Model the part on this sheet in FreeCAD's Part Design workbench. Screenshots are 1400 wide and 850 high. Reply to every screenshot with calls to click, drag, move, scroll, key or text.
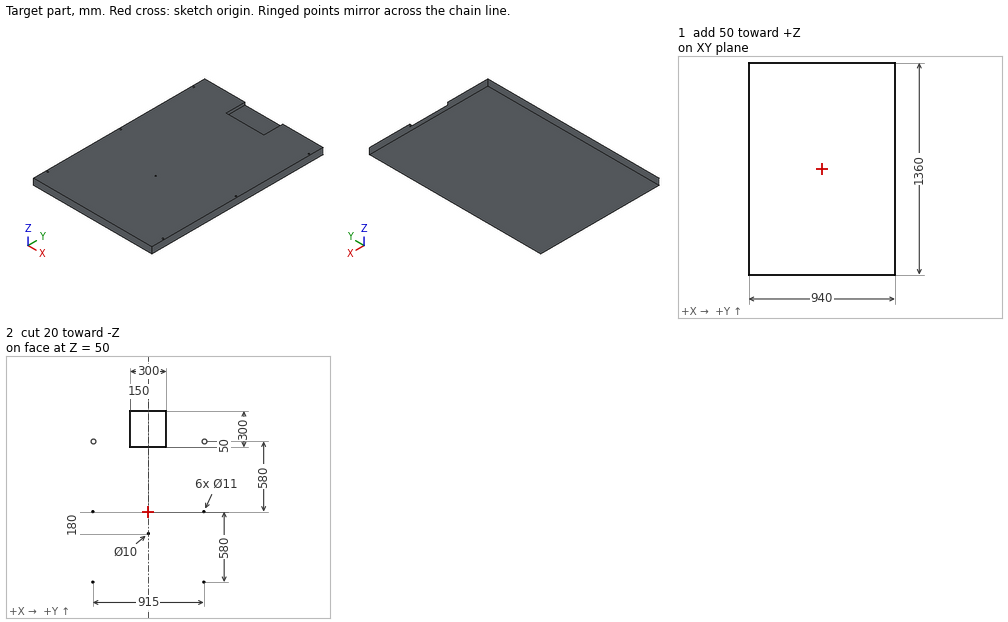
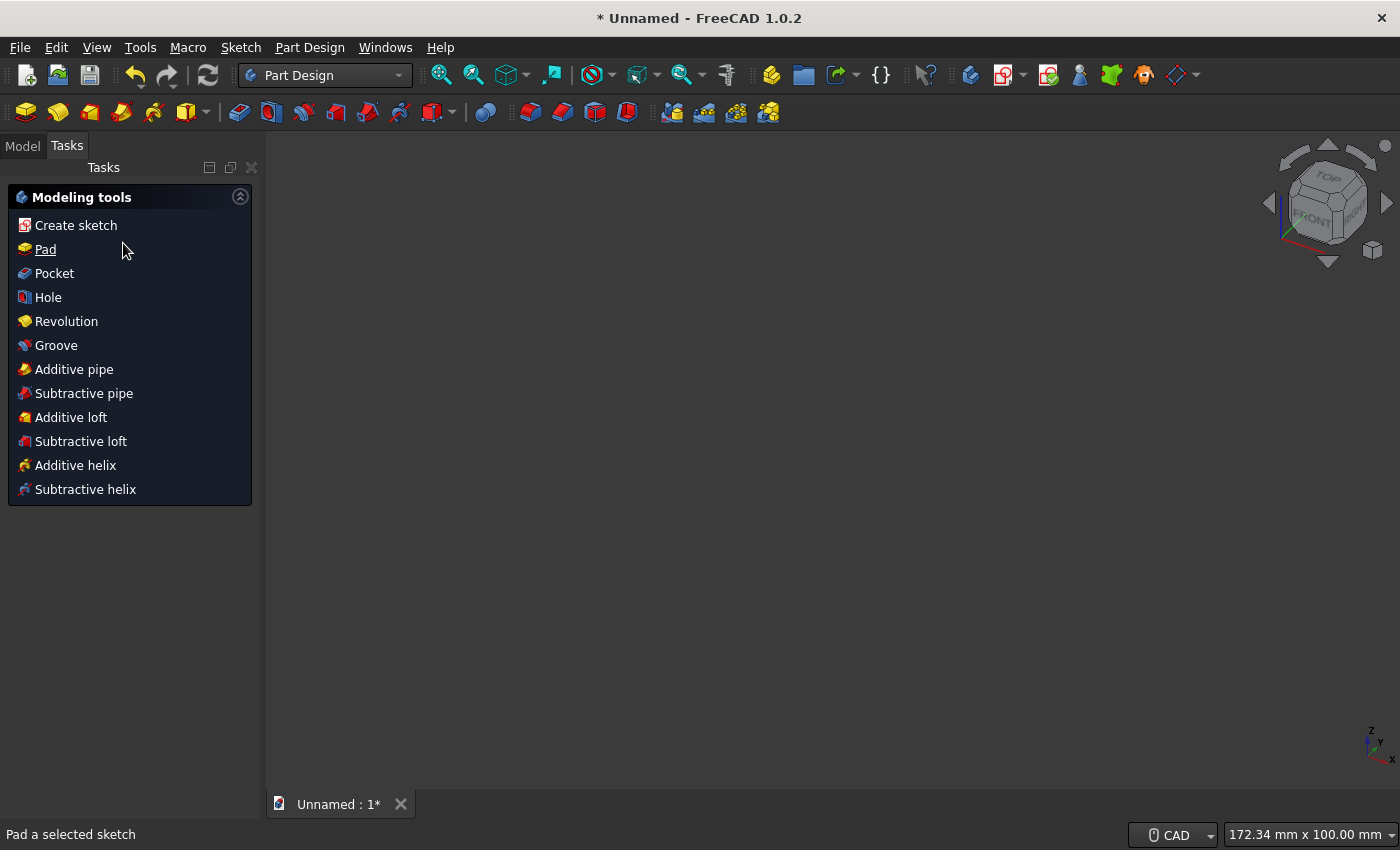
click(26, 112)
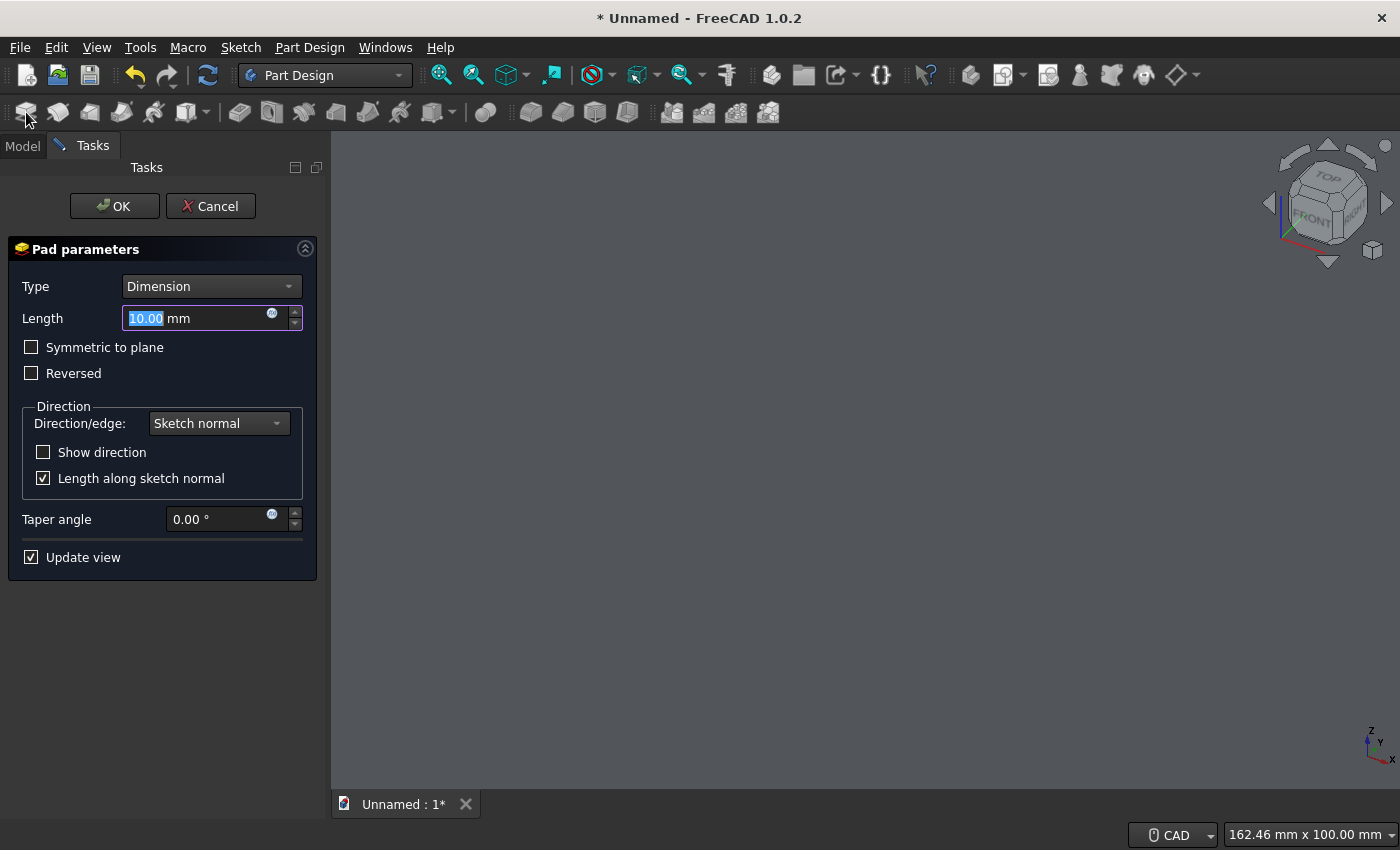
text(50)
key(Tab)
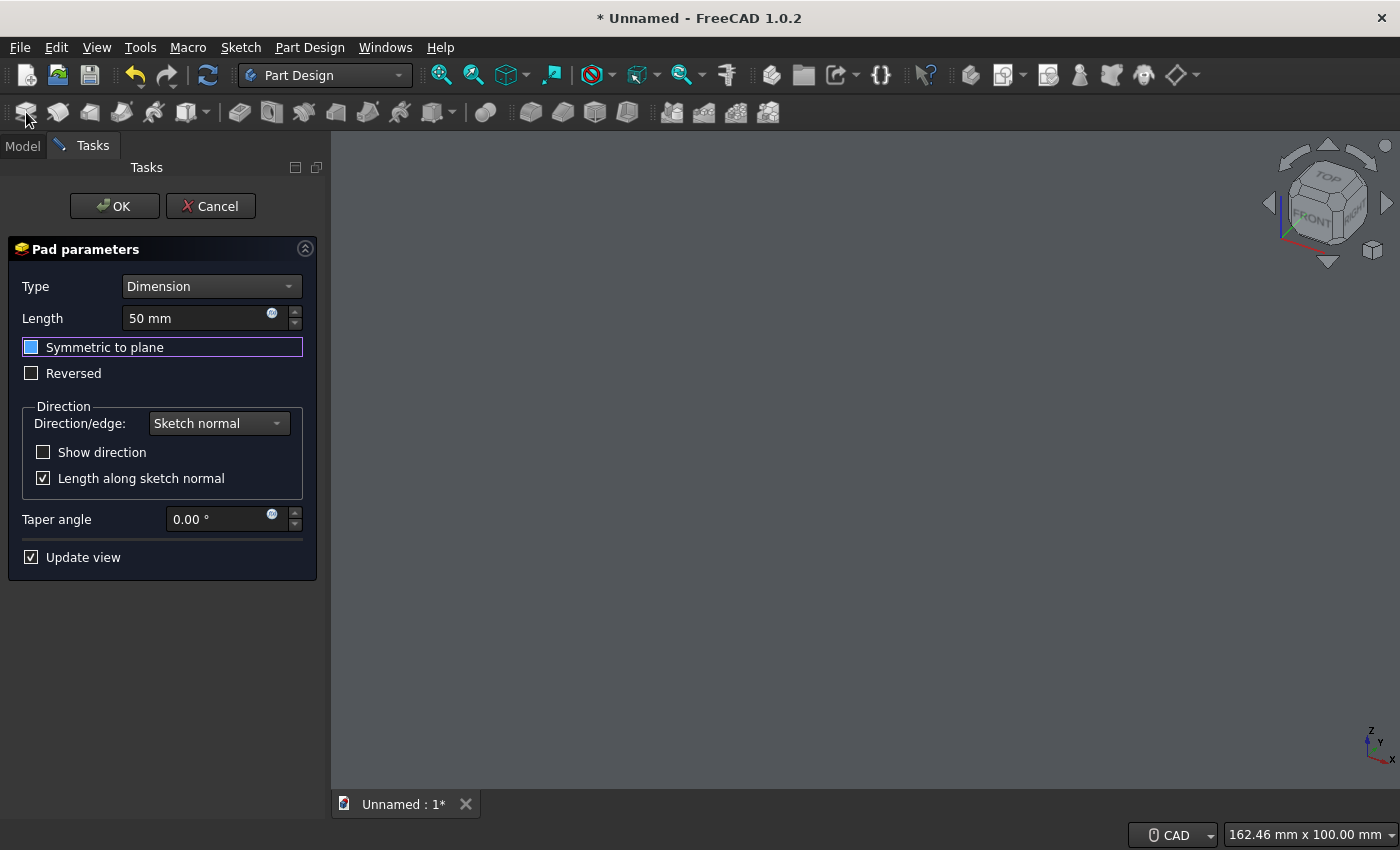
click(115, 206)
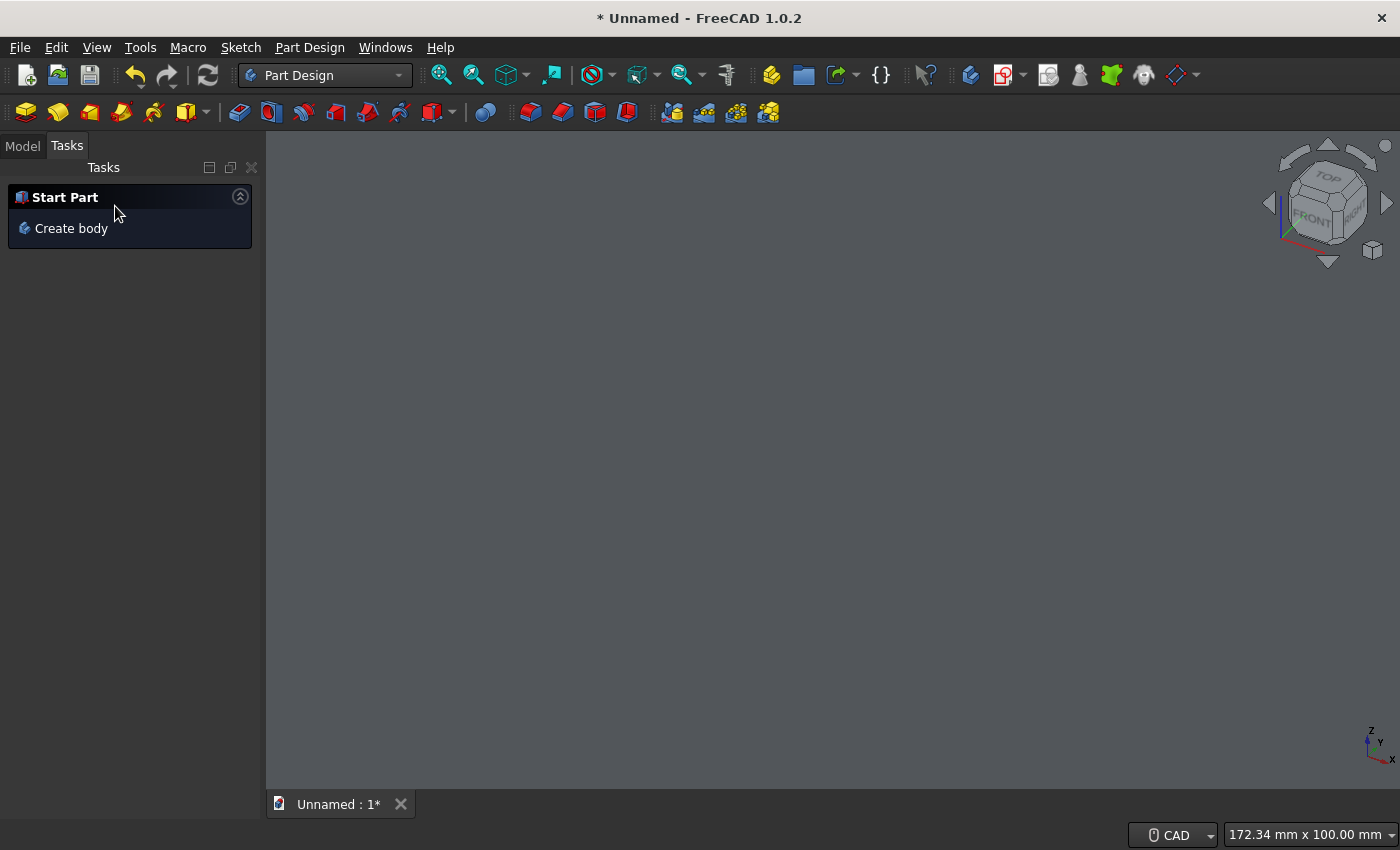
key(v)
key(f)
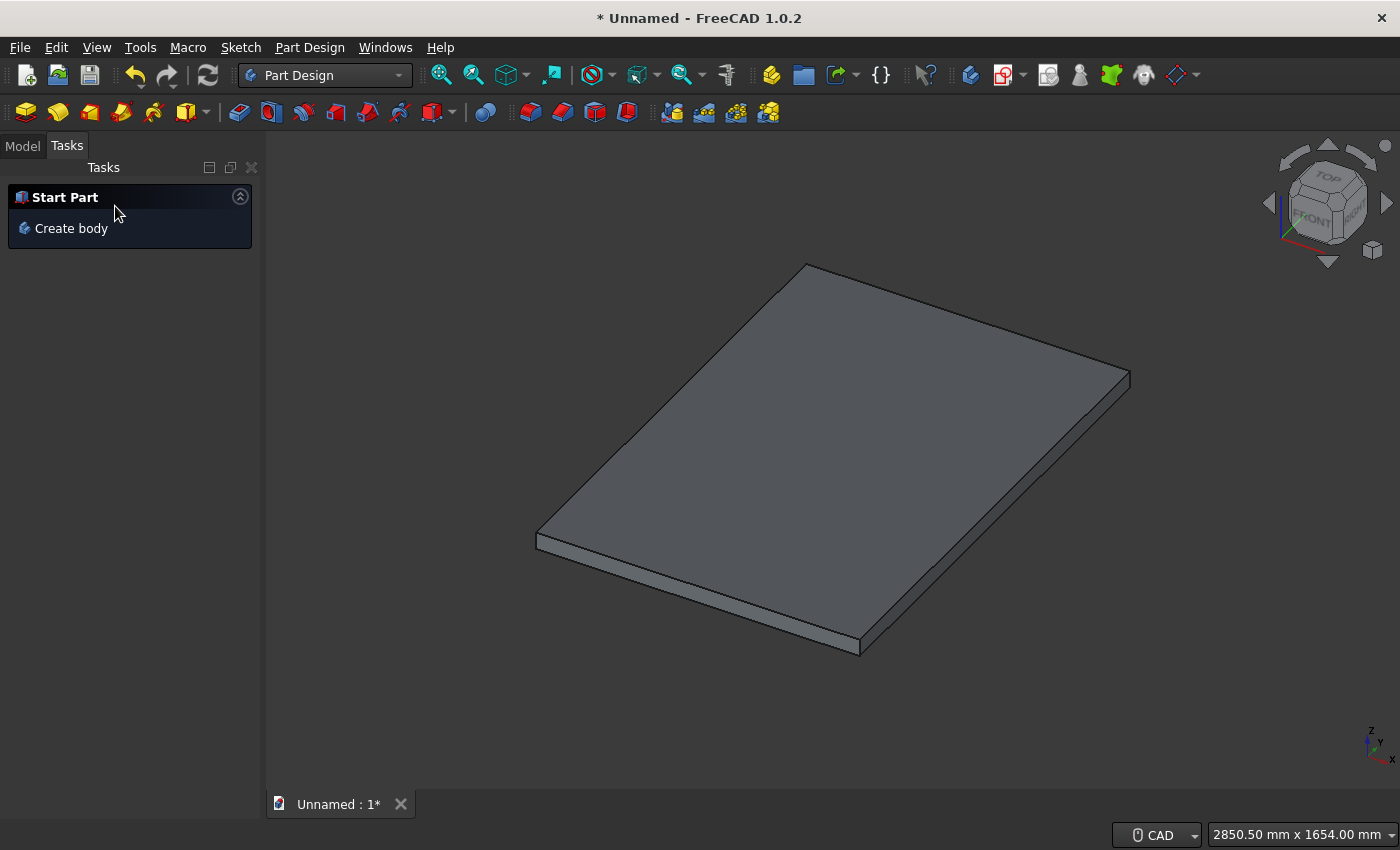
click(872, 412)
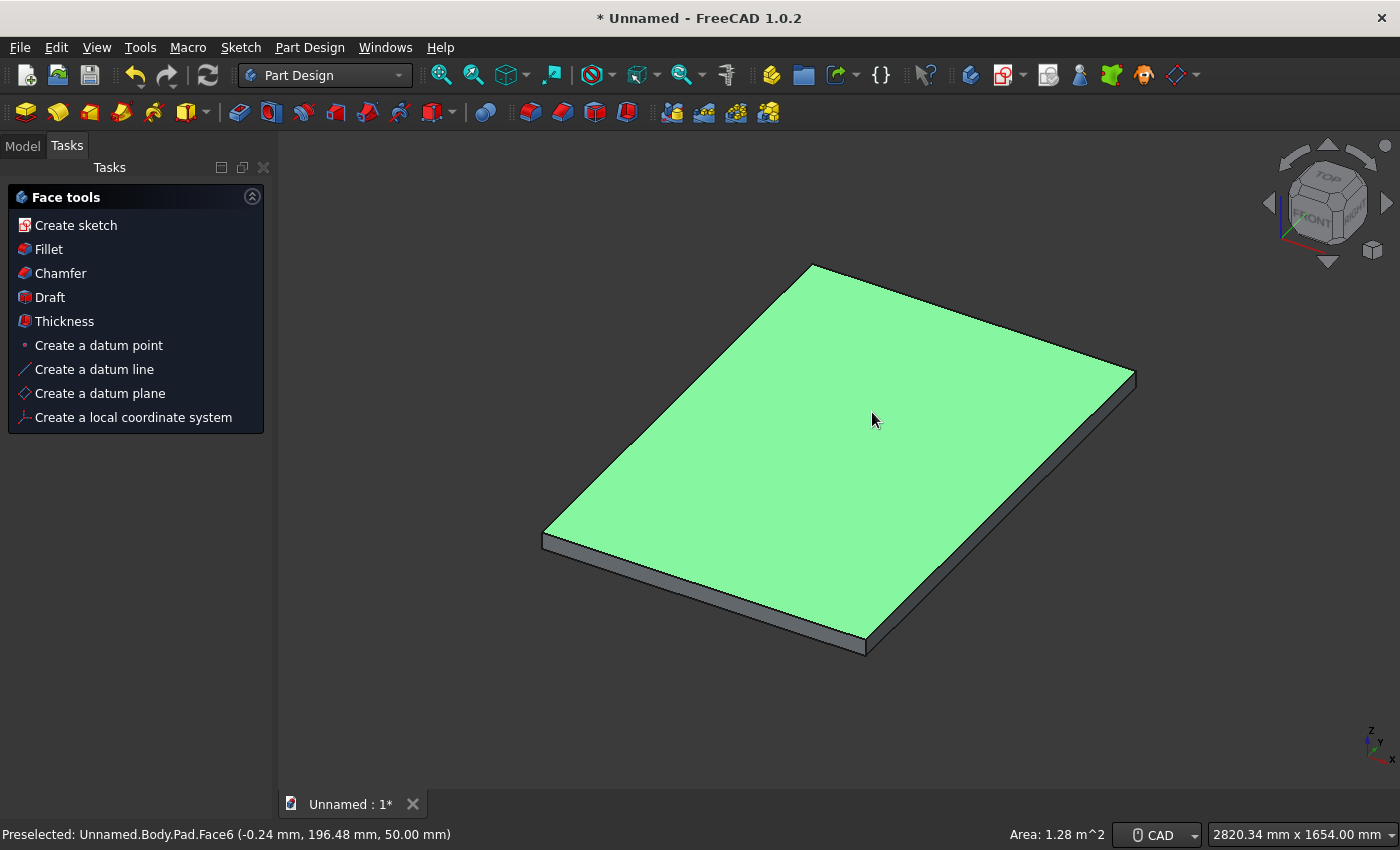
click(1004, 76)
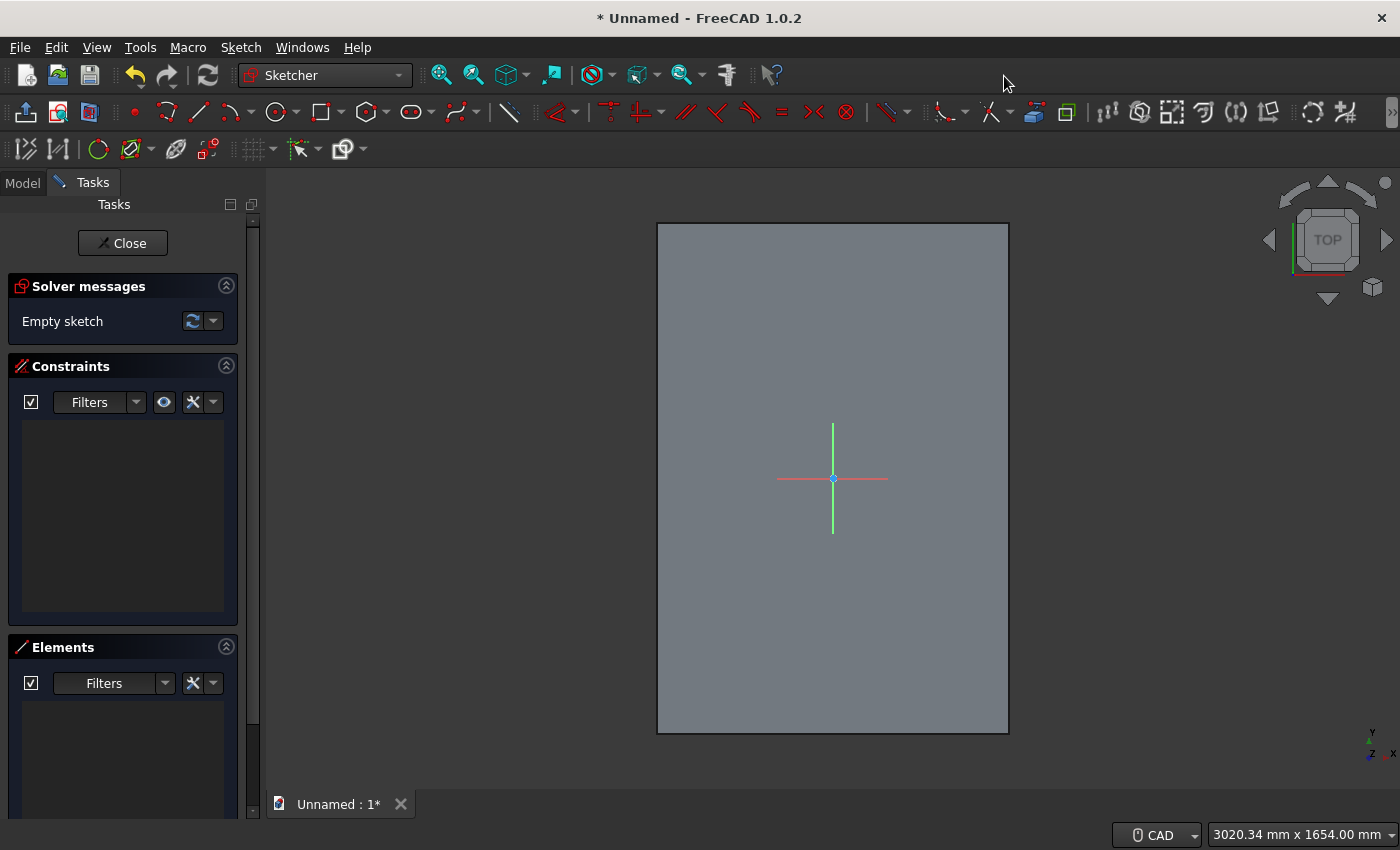
scroll(455, 686, down, 1)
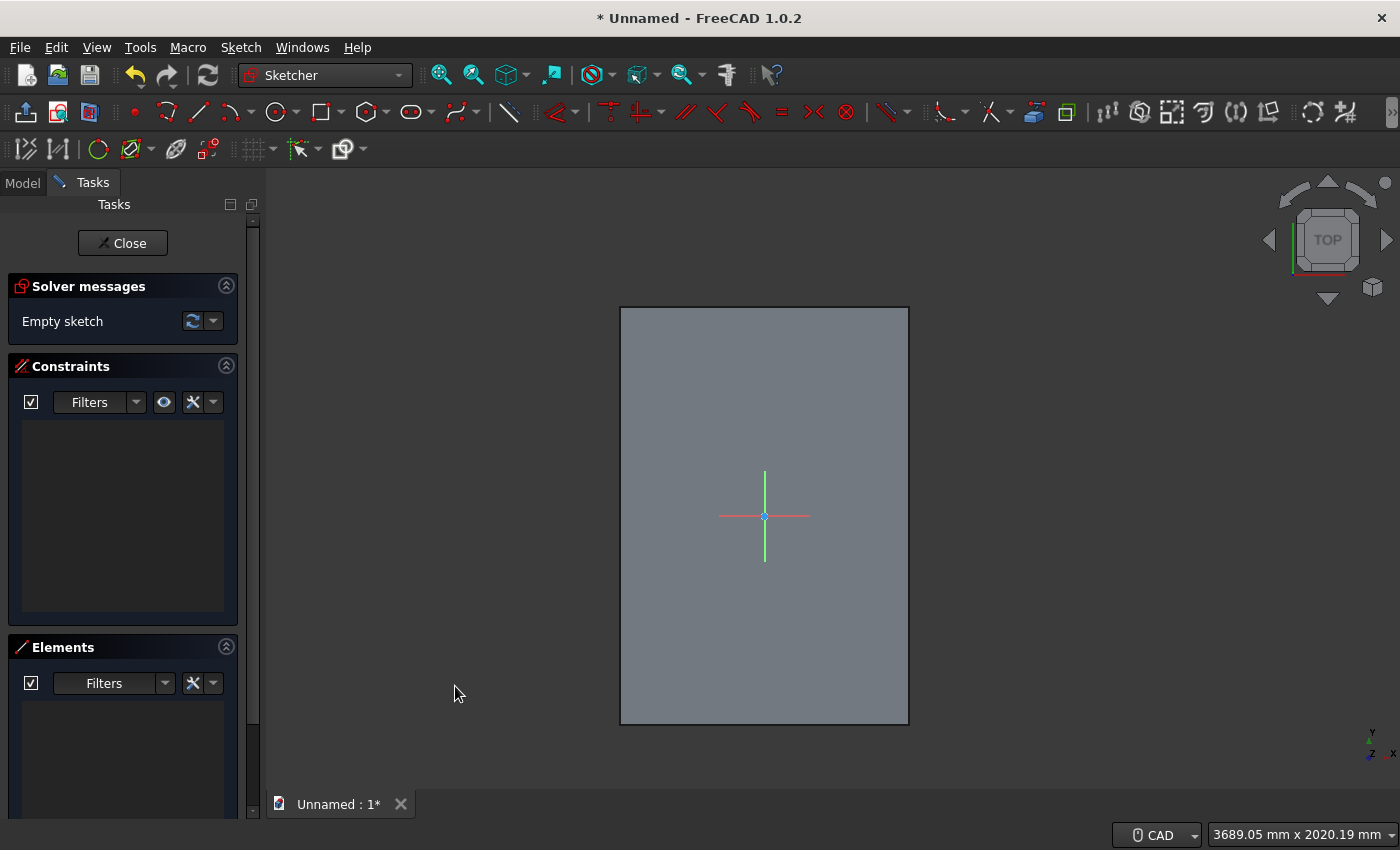
key(g)
key(r)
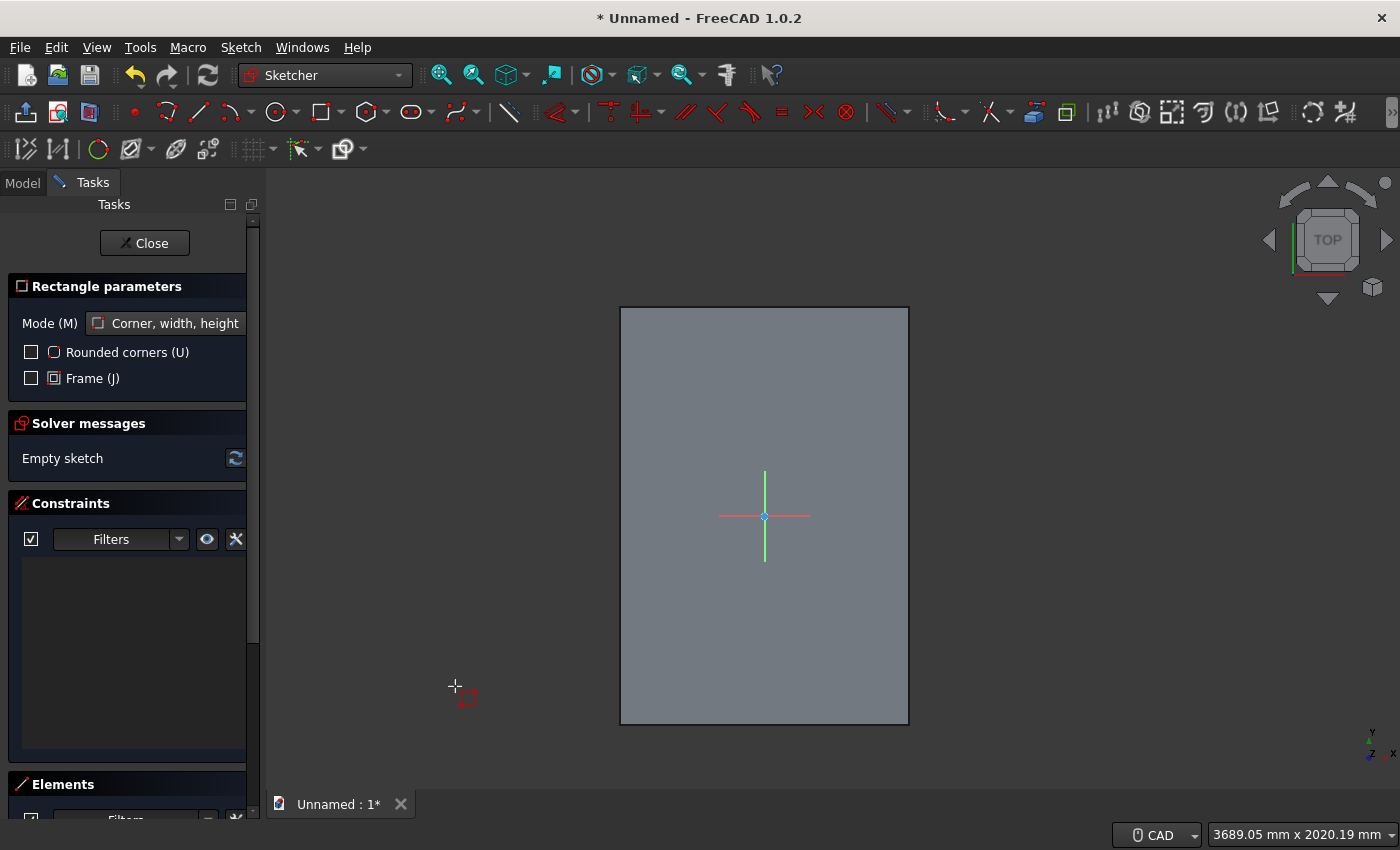
click(718, 261)
move(811, 353)